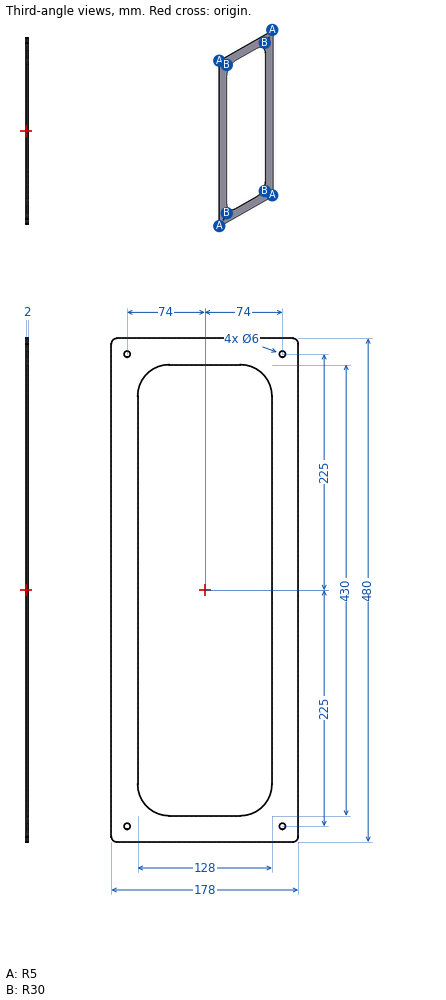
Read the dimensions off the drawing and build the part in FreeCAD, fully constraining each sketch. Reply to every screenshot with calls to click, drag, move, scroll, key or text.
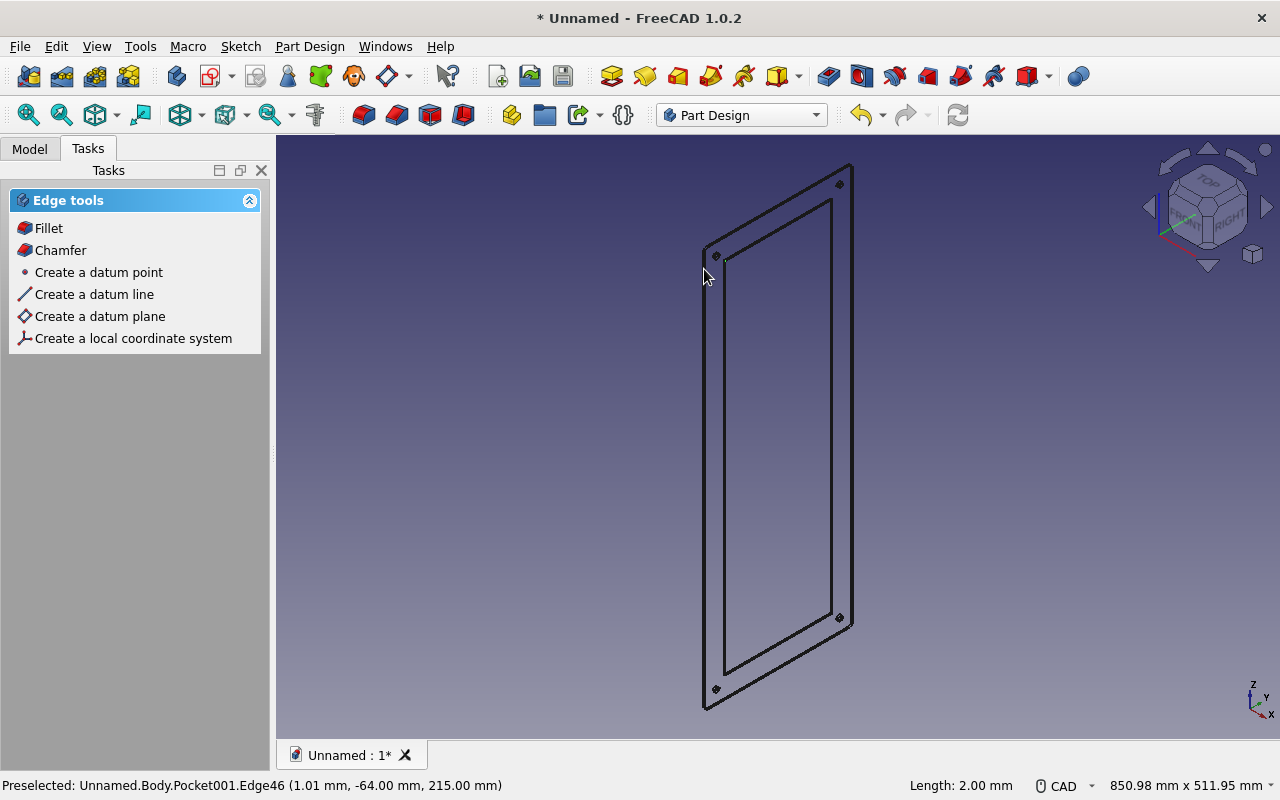
key(2)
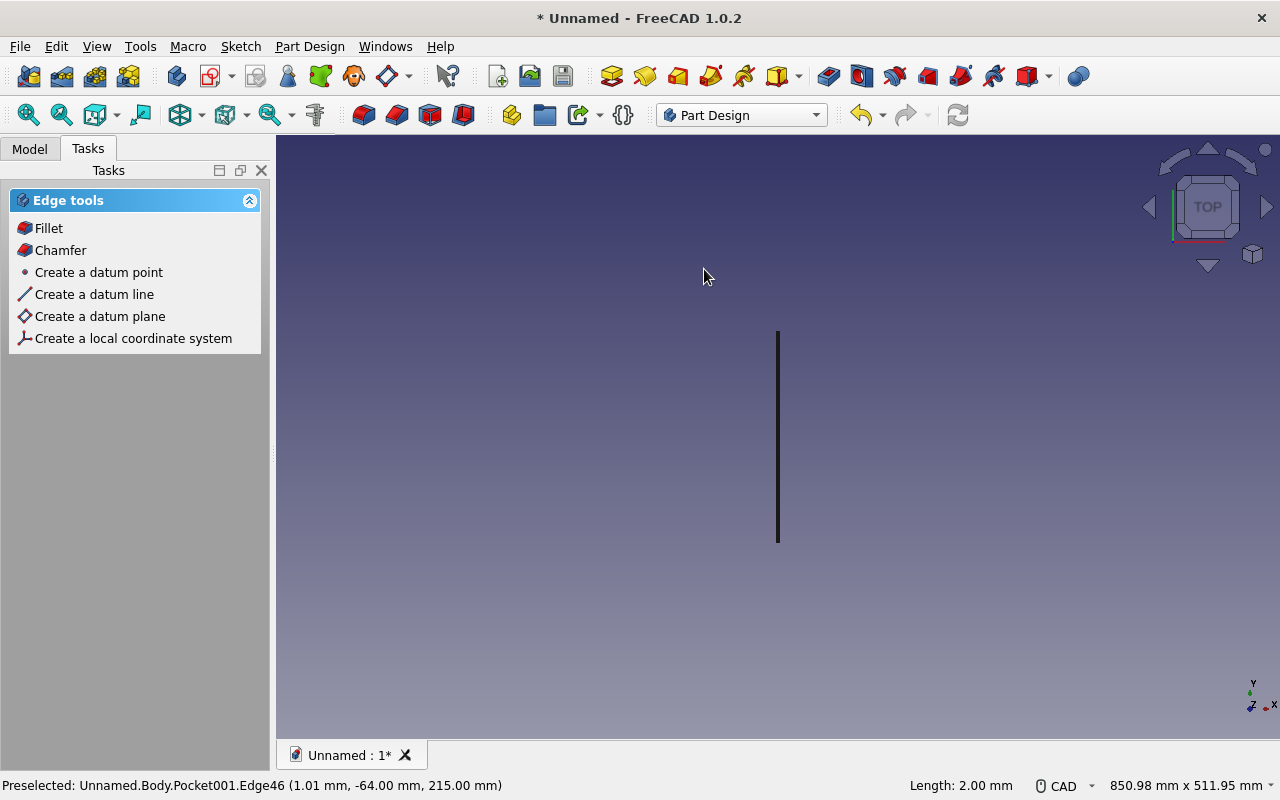
key(v)
key(f)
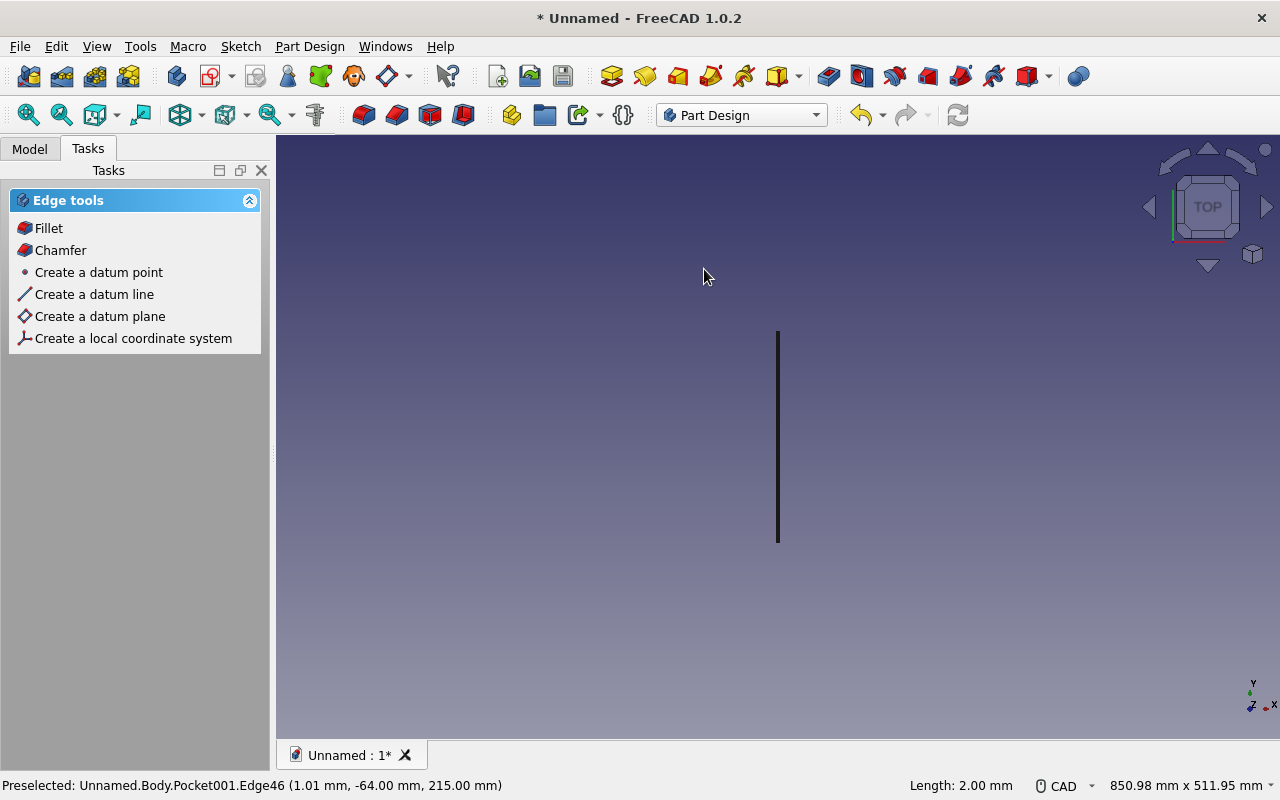
scroll(778, 360, up, 15)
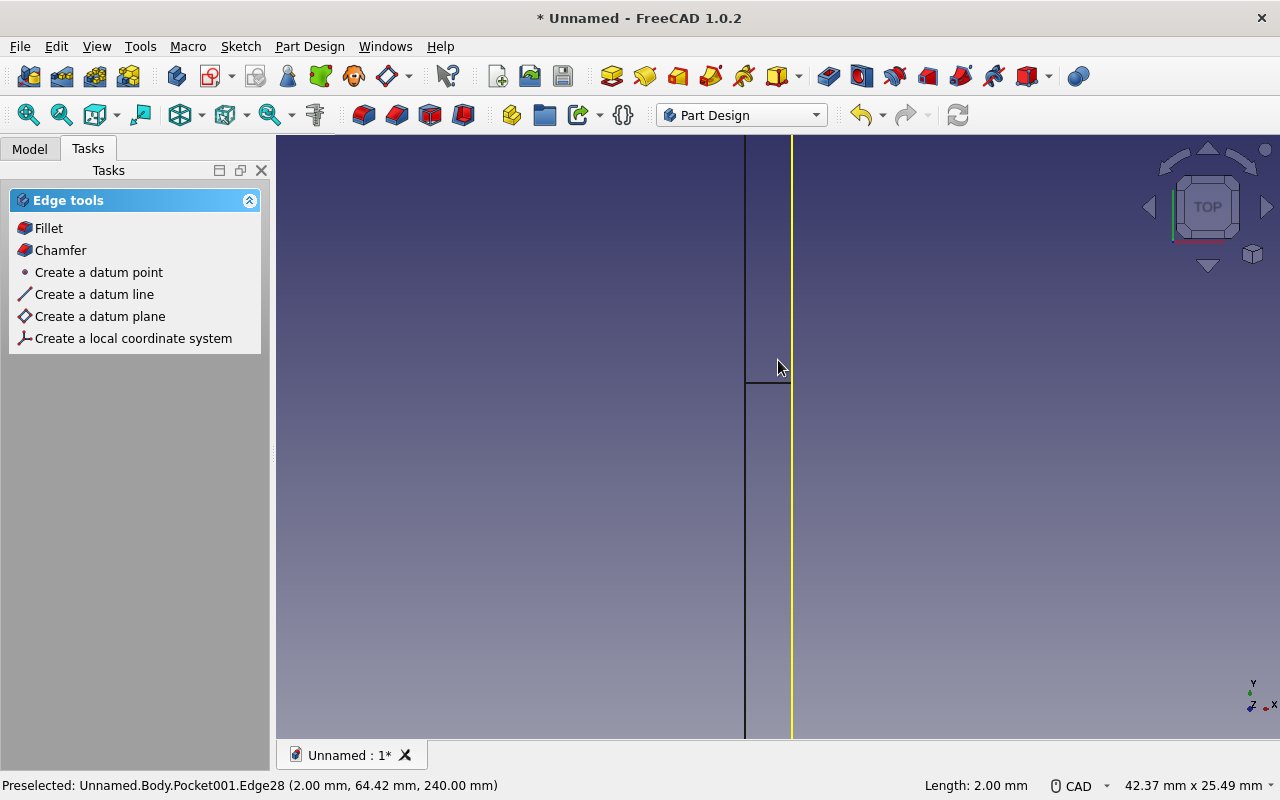
click(768, 382, ctrl)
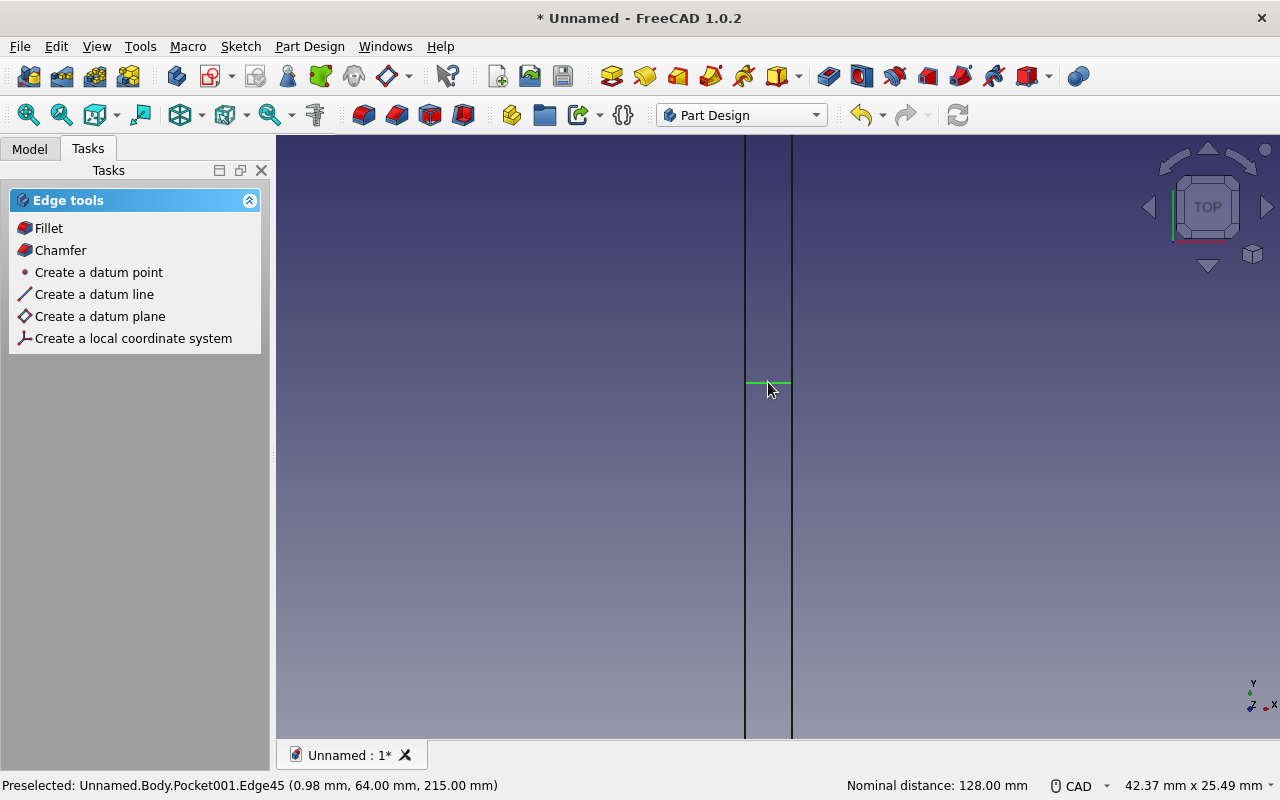
key(v)
key(f)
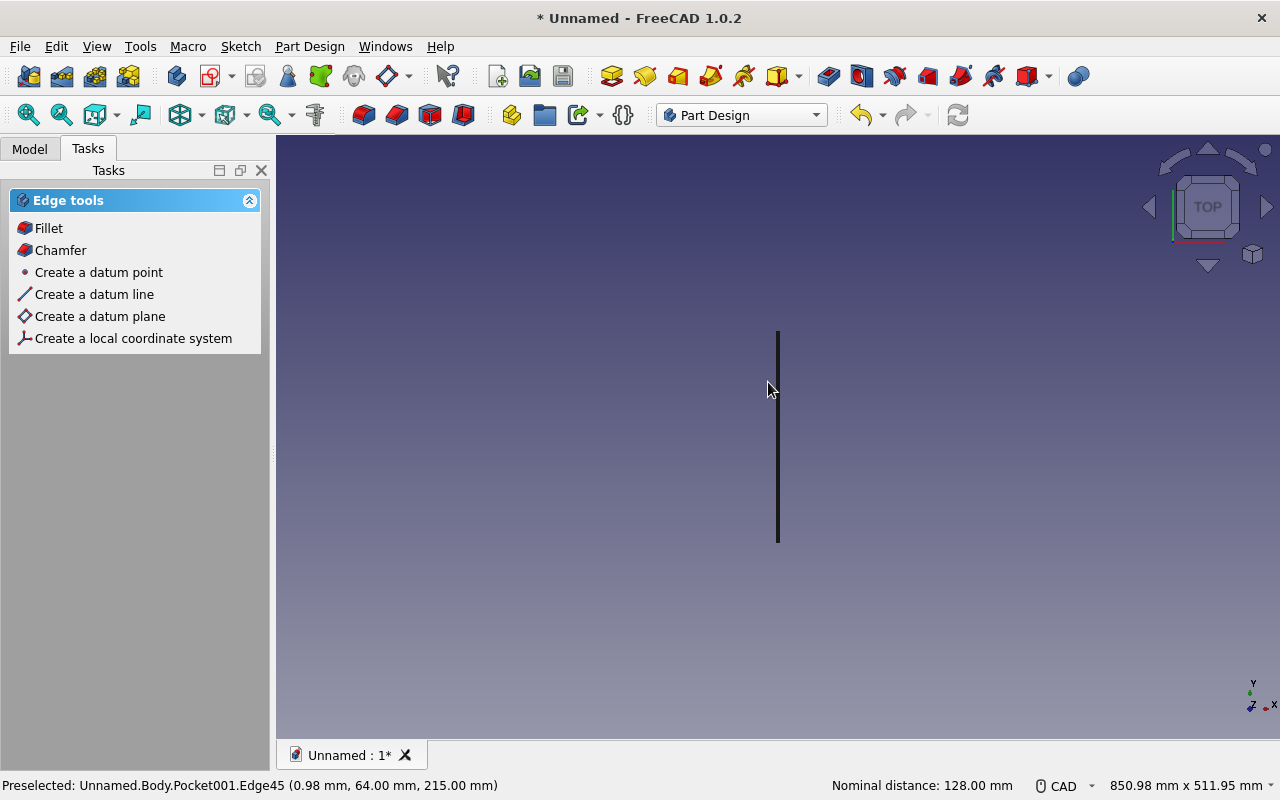
key(1)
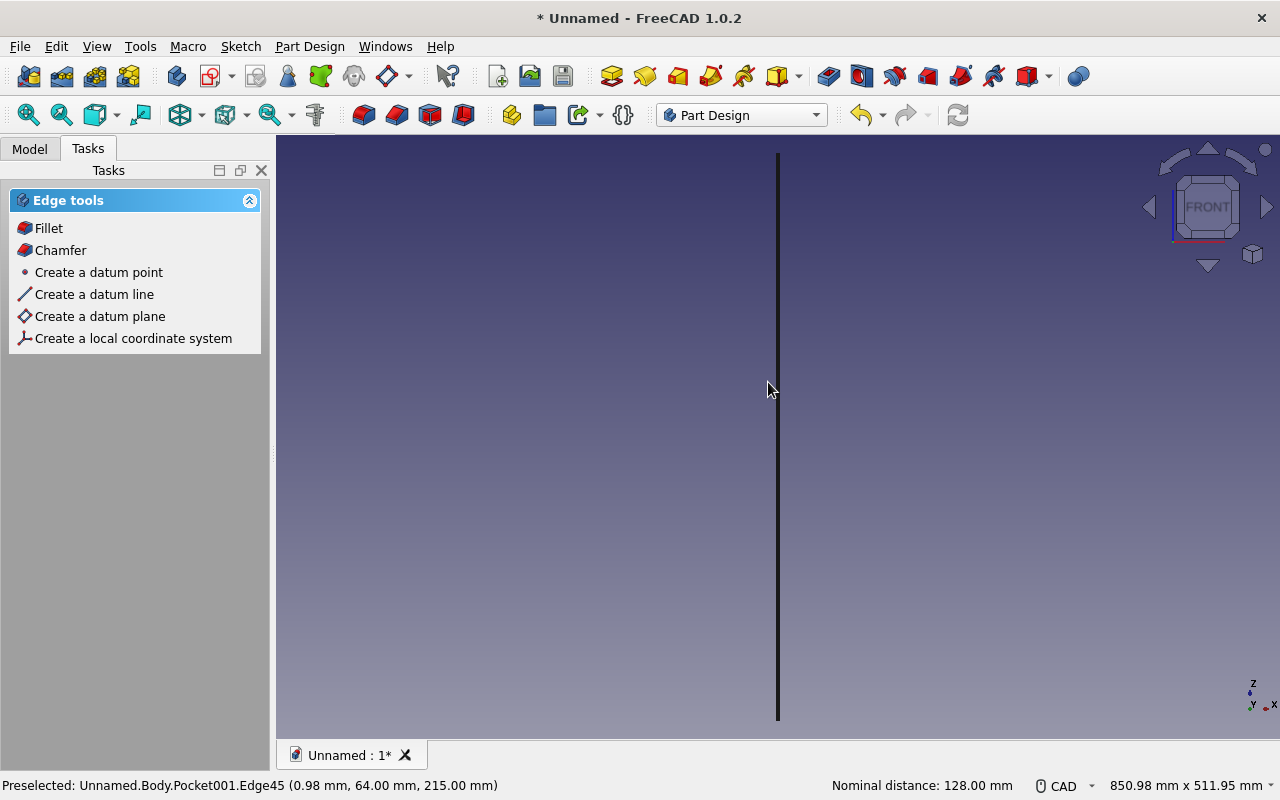
scroll(778, 690, up, 15)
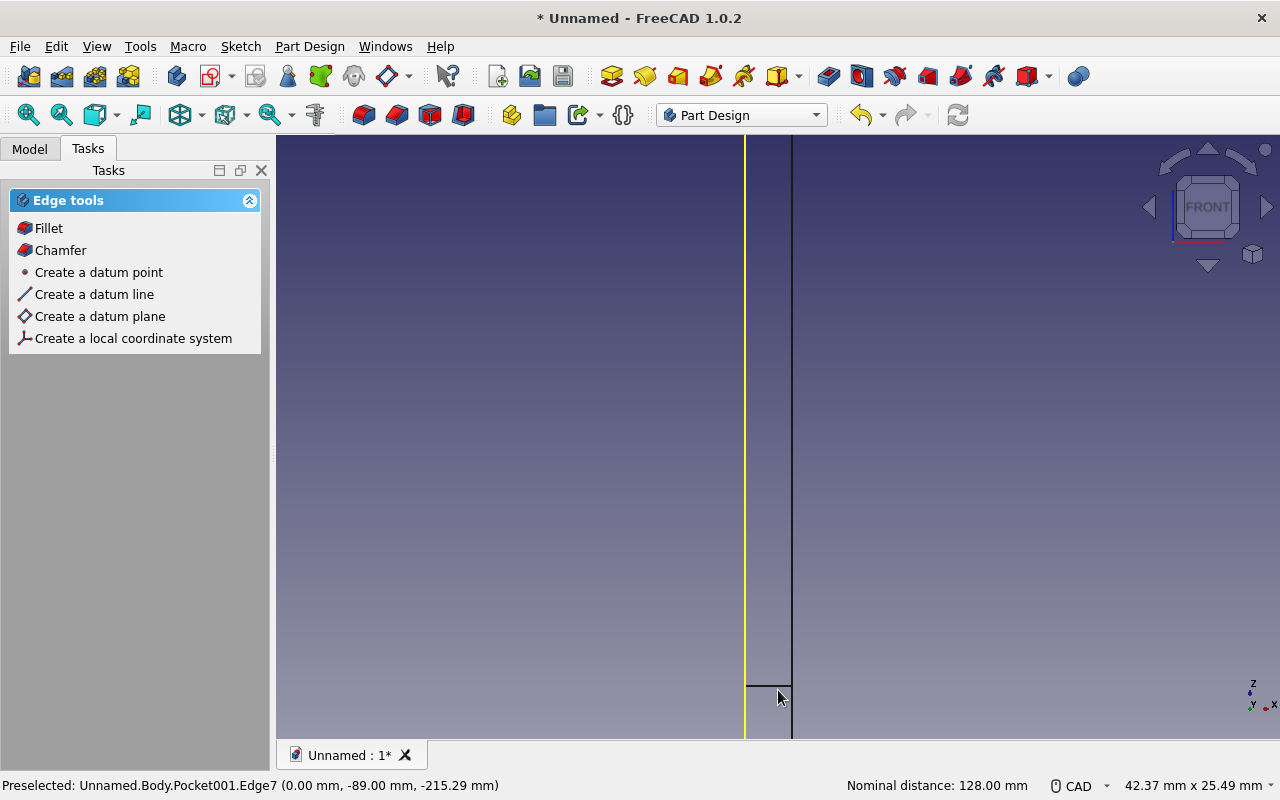
click(768, 685, ctrl)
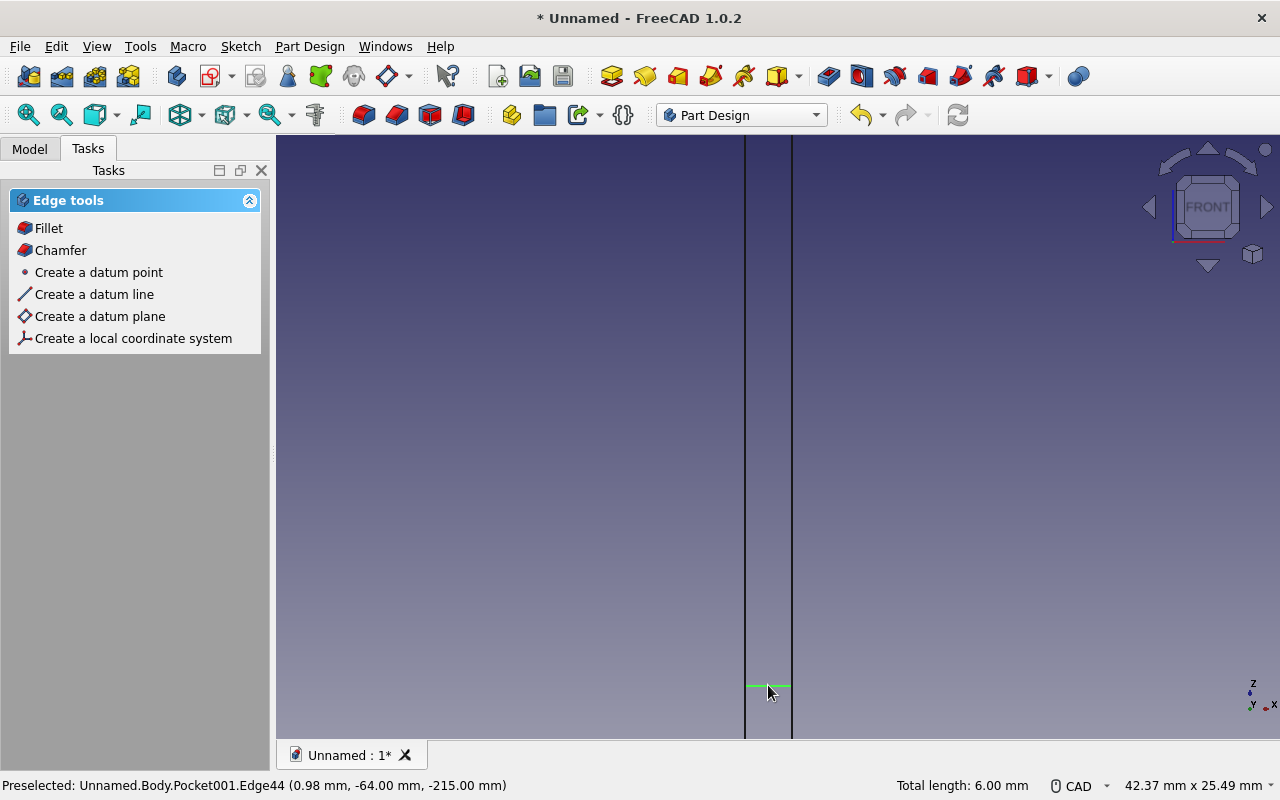
click(29, 116)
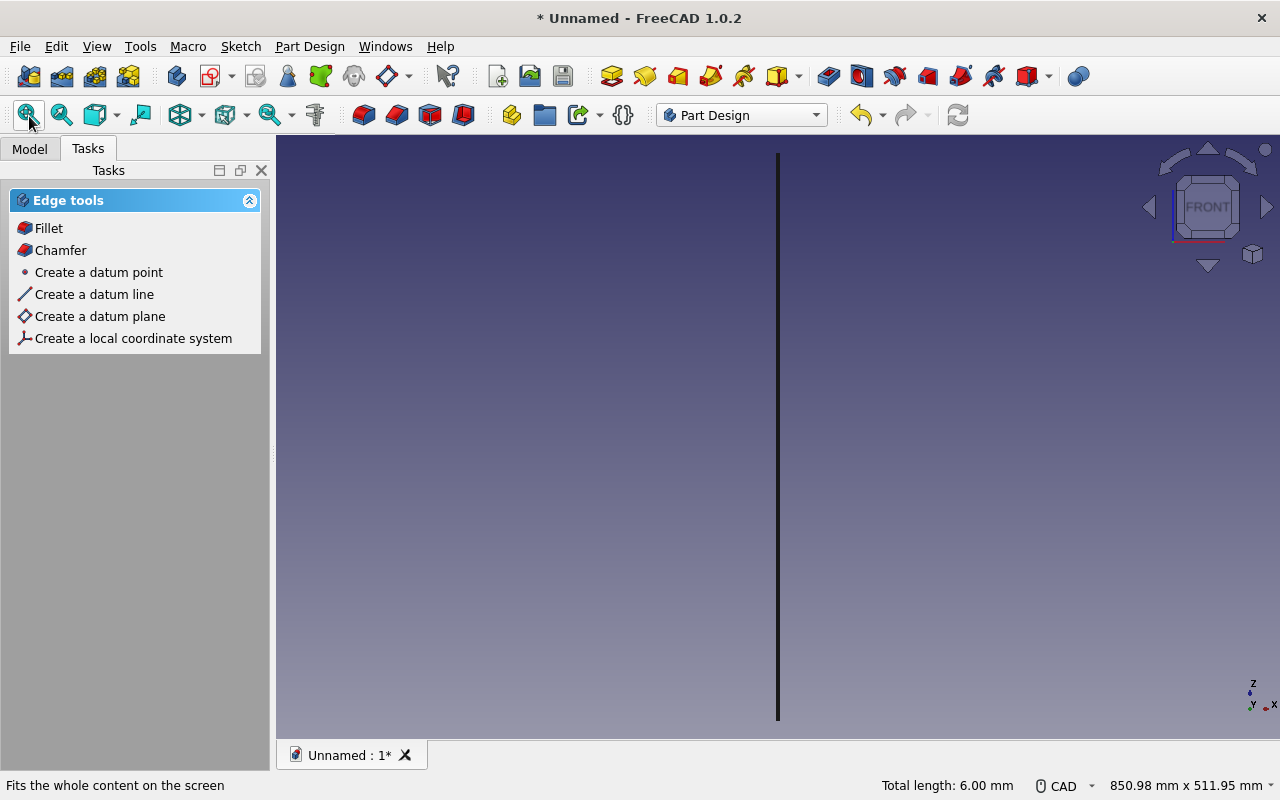
key(3)